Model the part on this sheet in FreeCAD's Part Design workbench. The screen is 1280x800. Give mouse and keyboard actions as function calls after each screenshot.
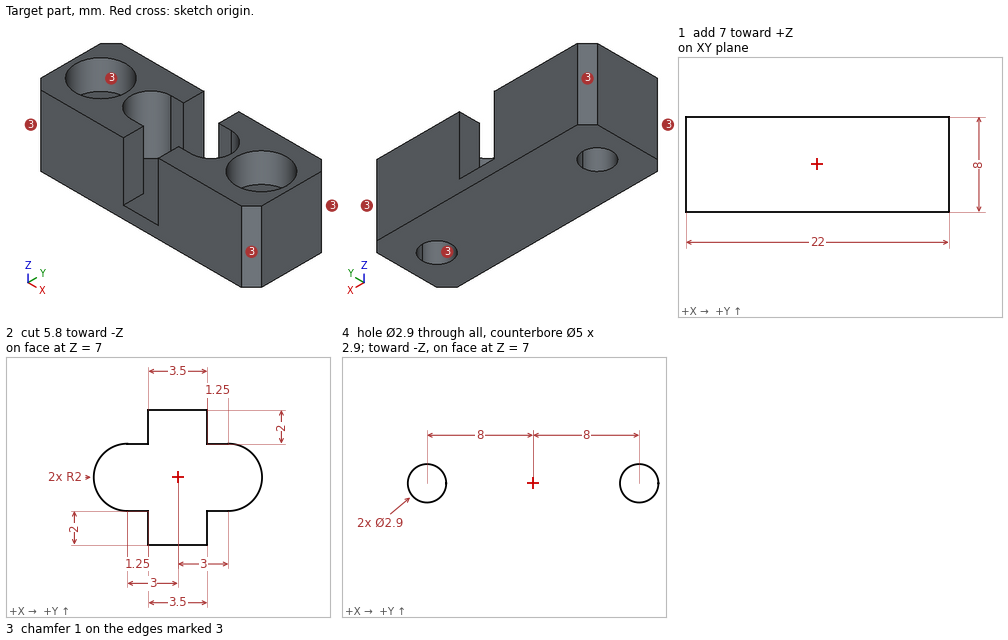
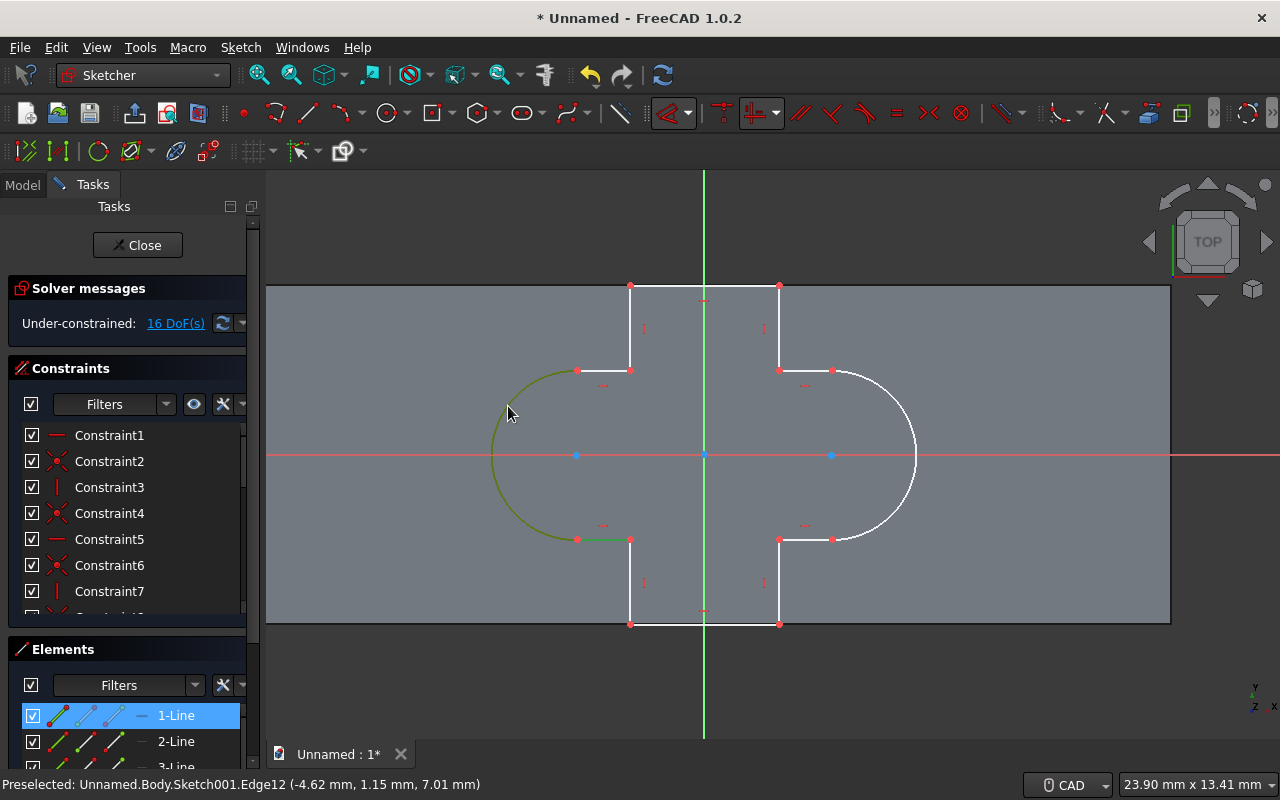
click(866, 114)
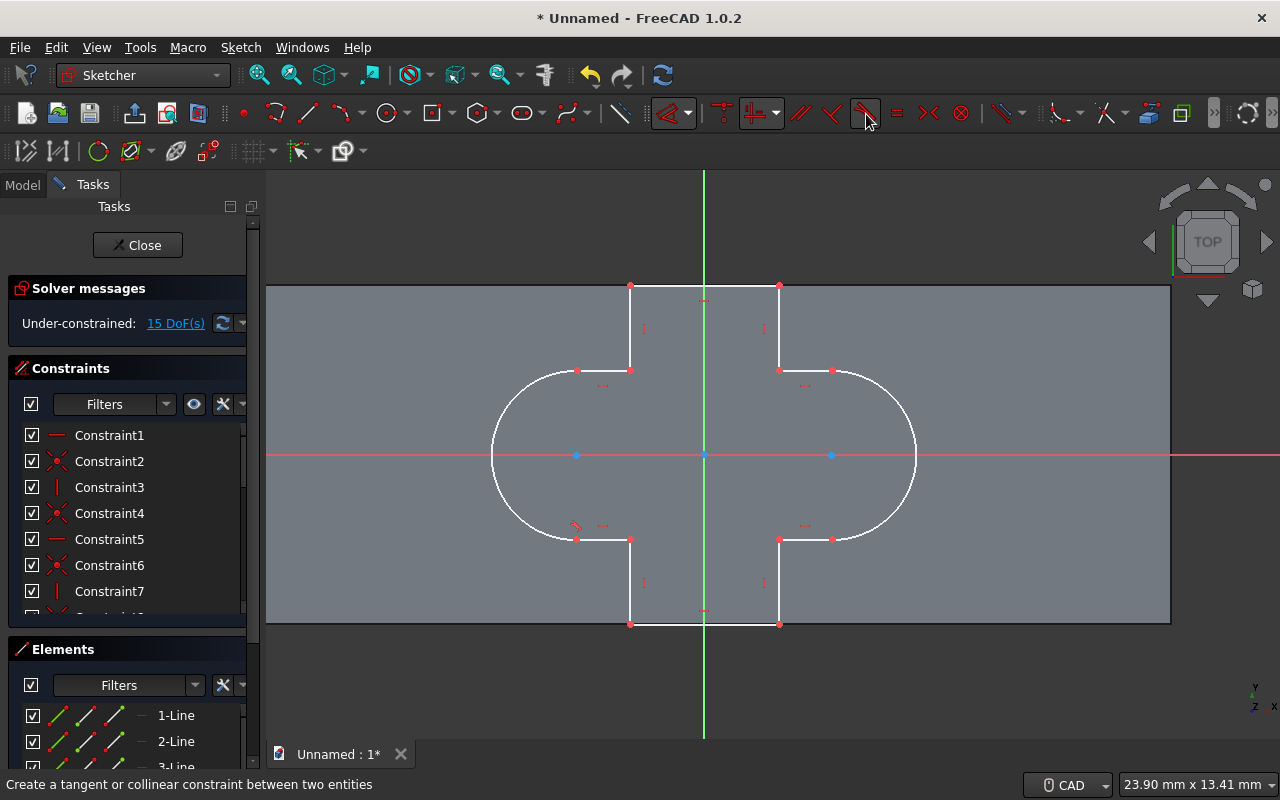
click(795, 540)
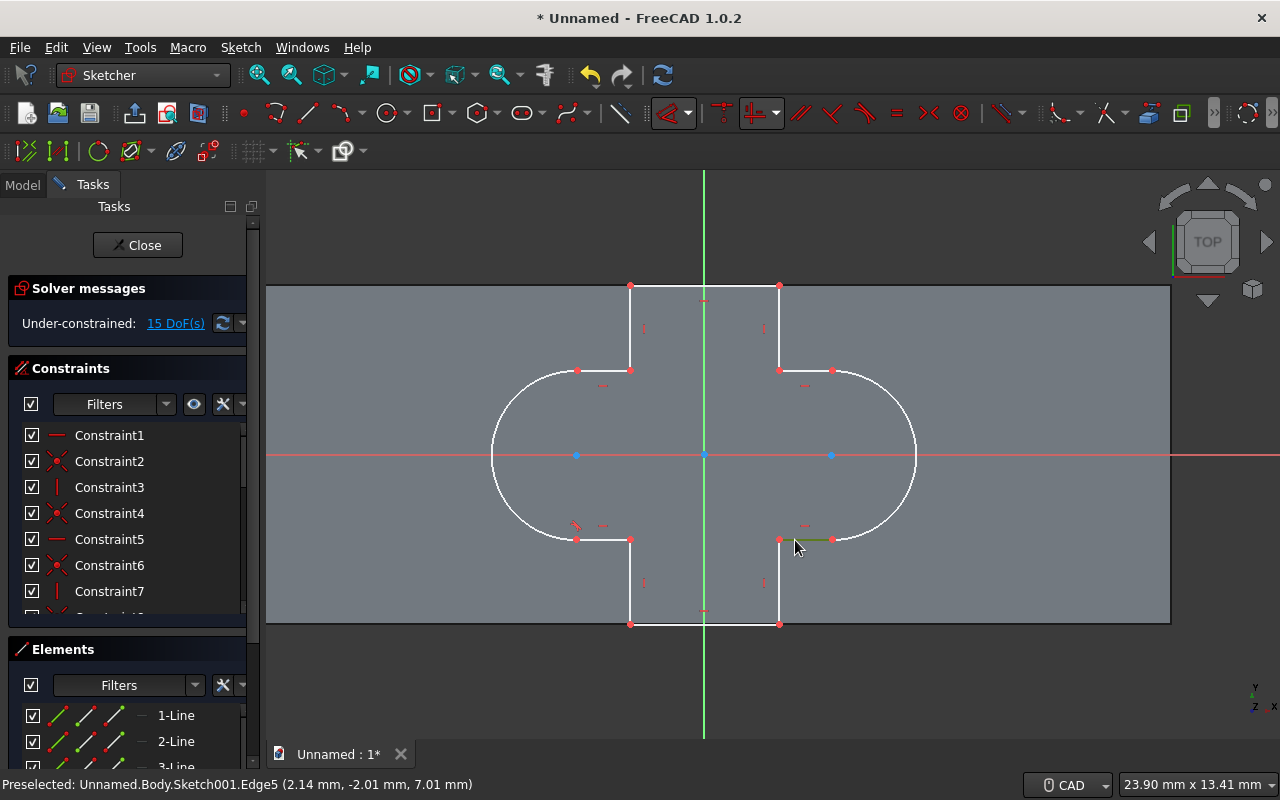
click(900, 505)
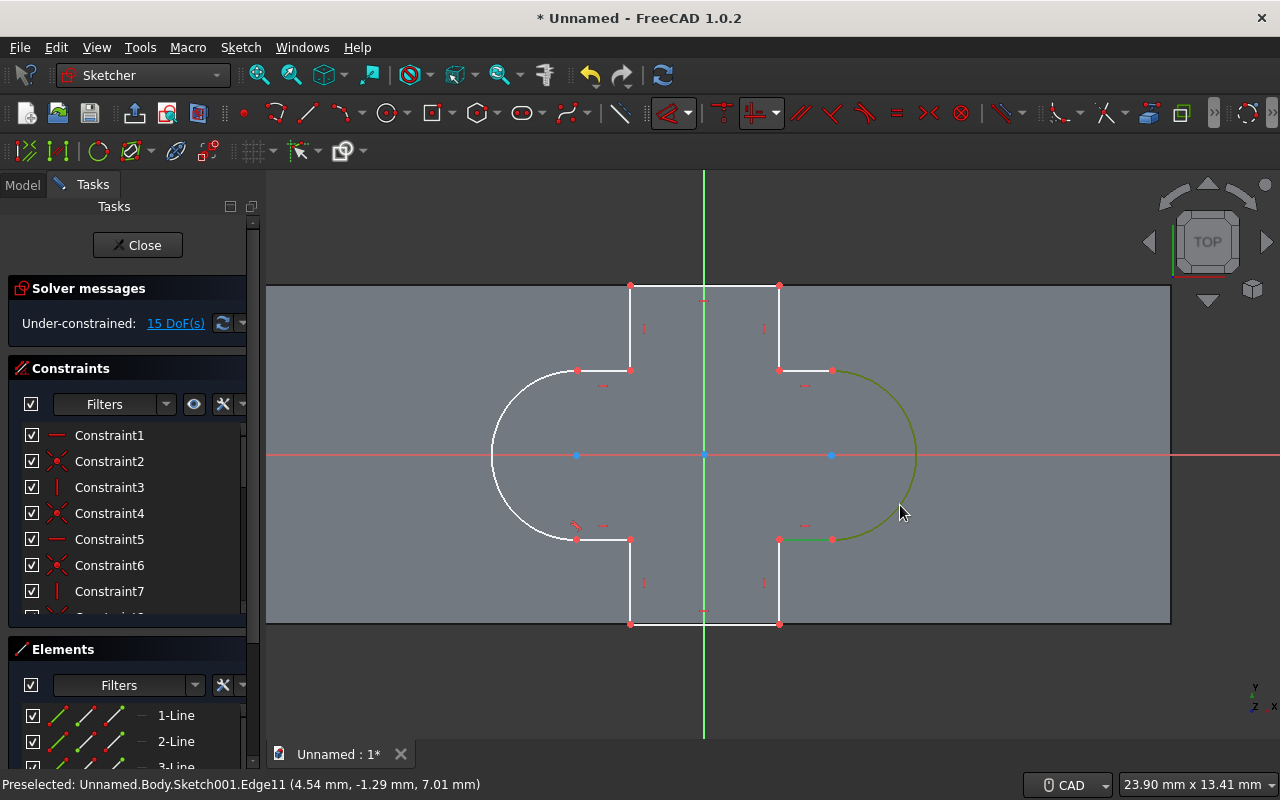
click(866, 114)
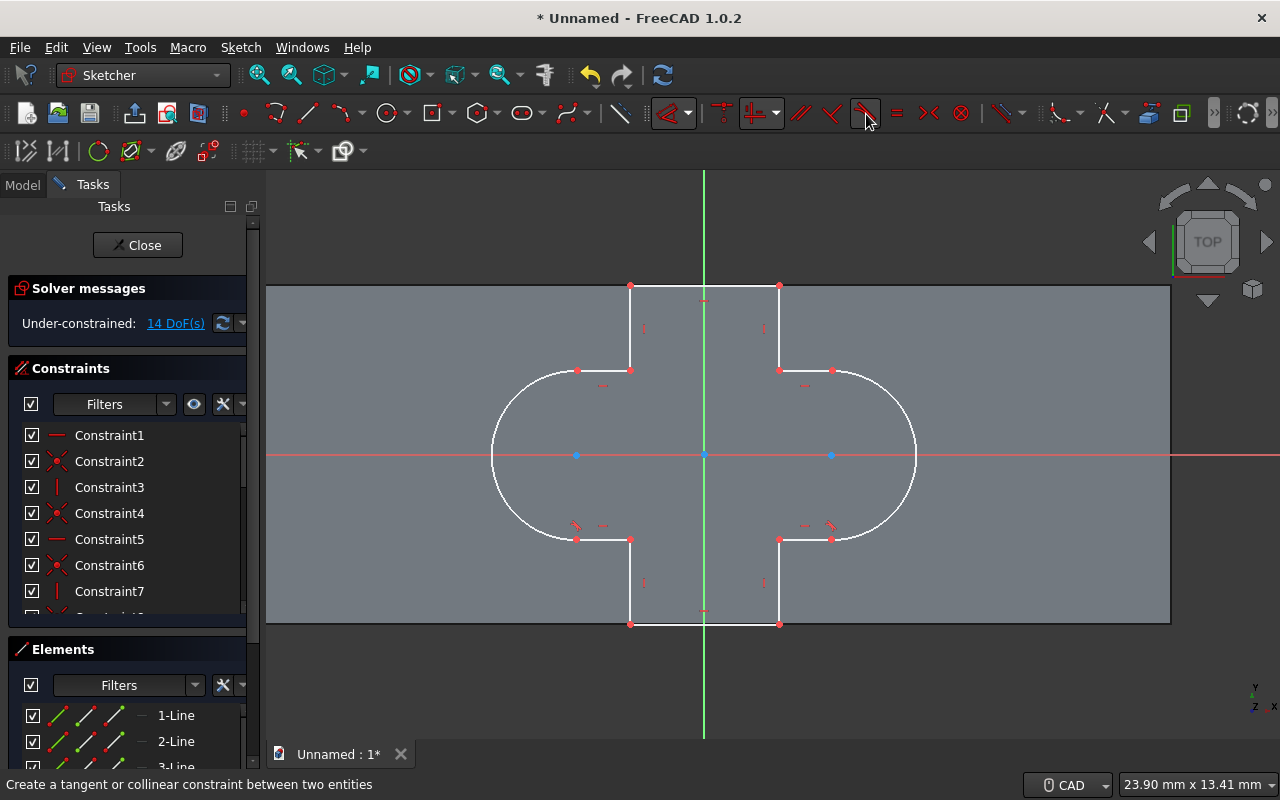
click(816, 371)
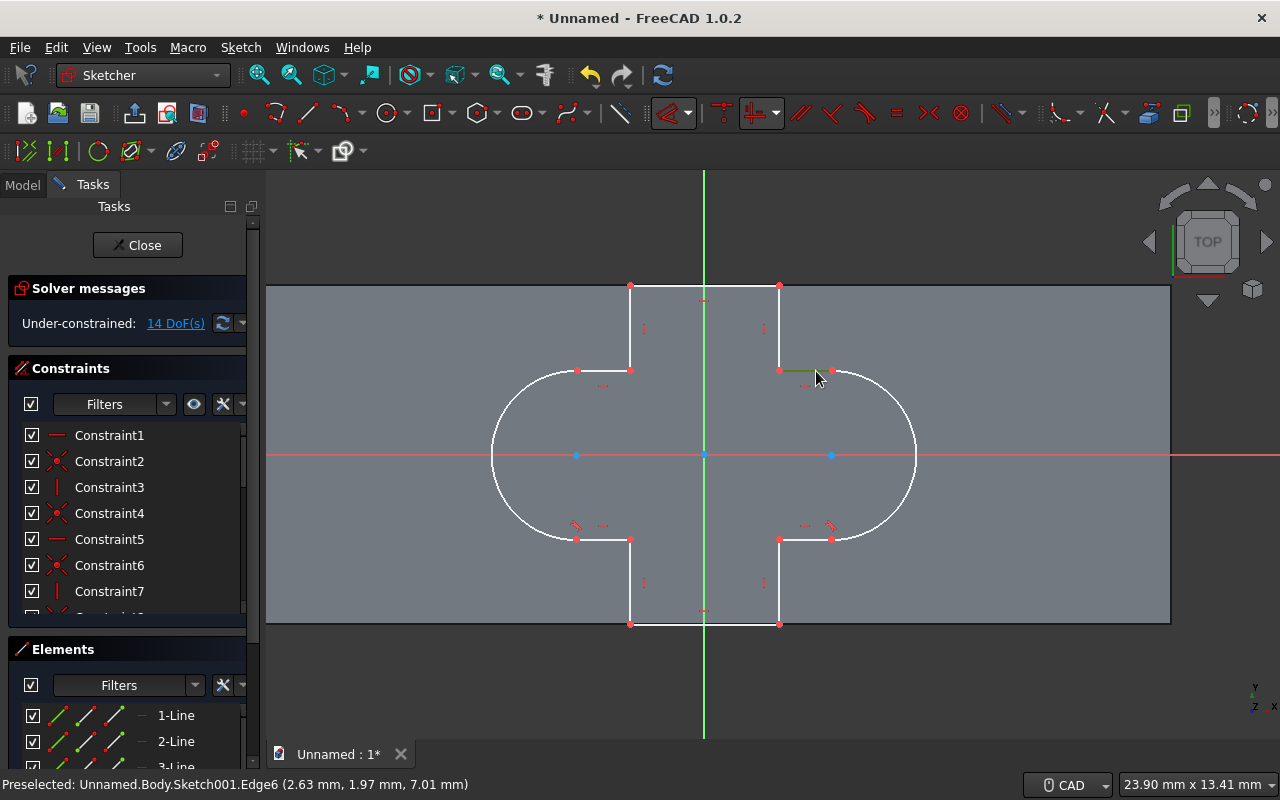
click(900, 505)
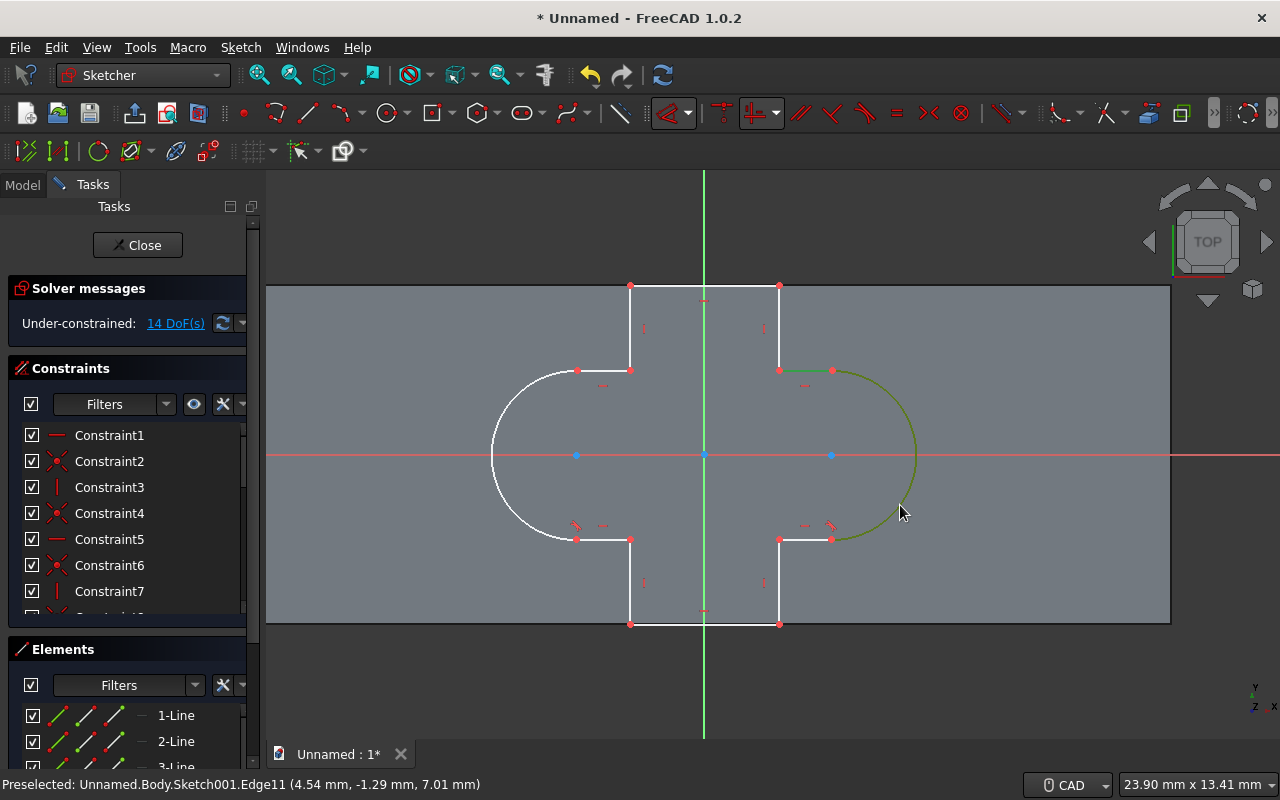
click(866, 114)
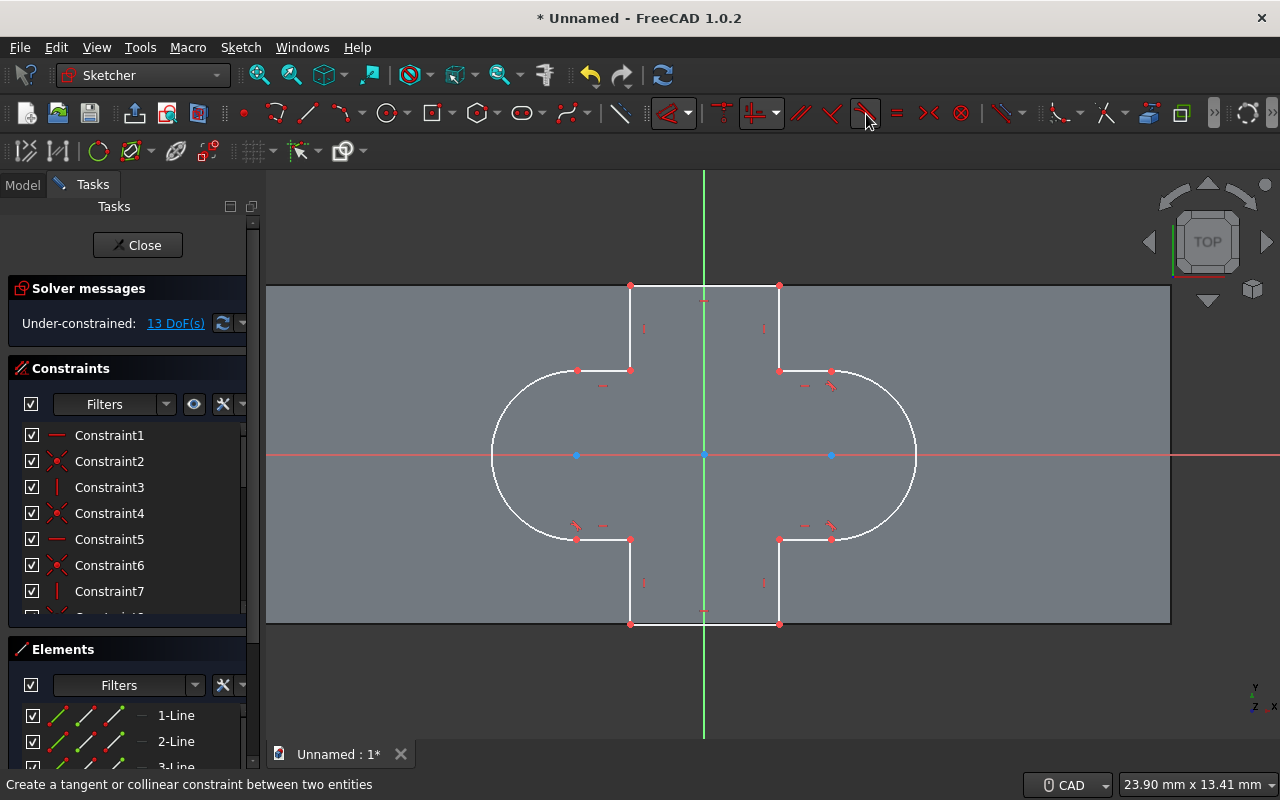
click(614, 371)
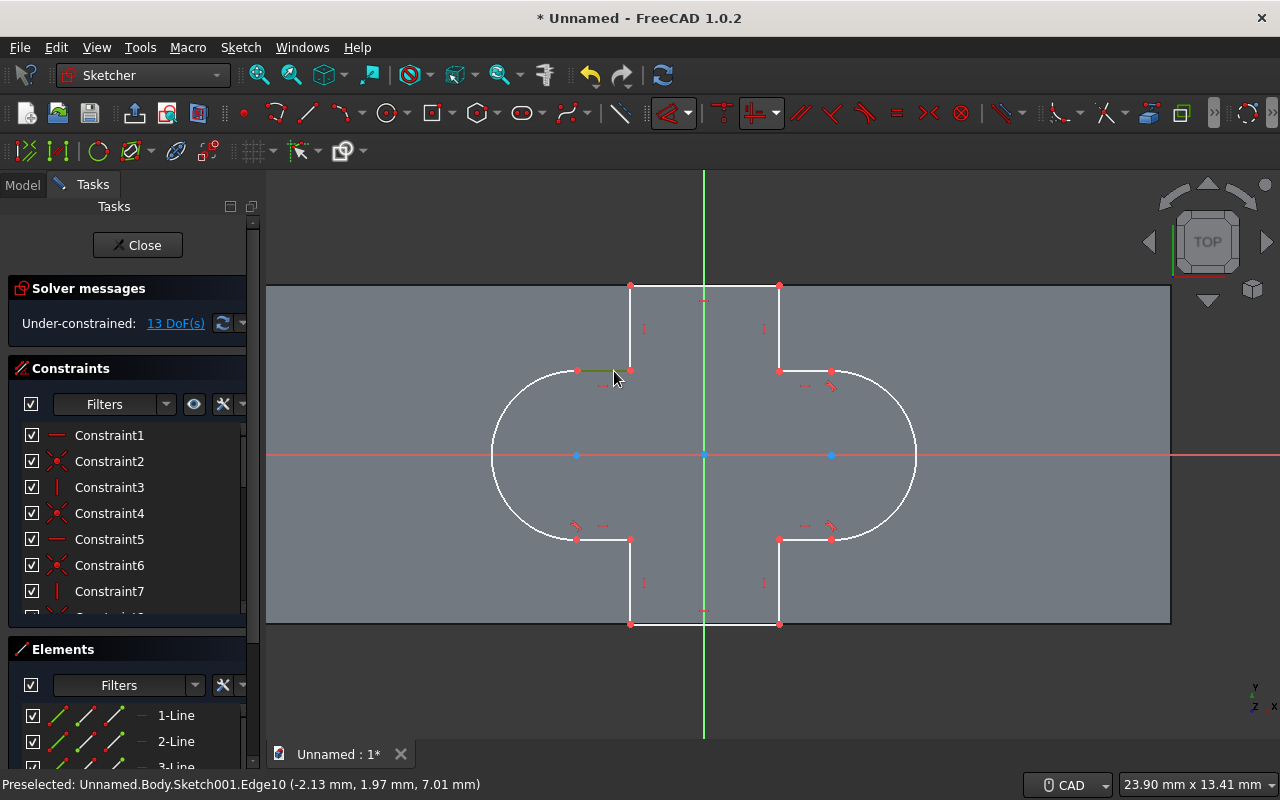
click(508, 405)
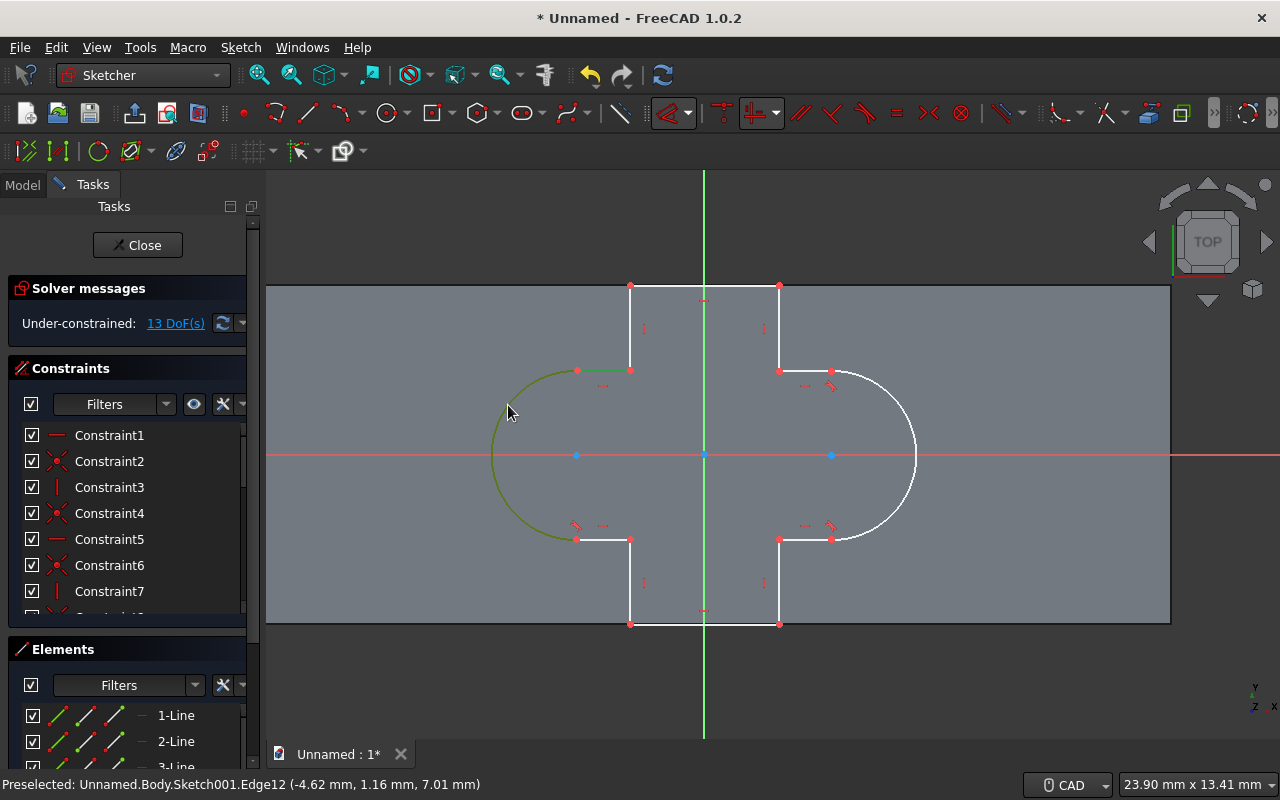
click(866, 114)